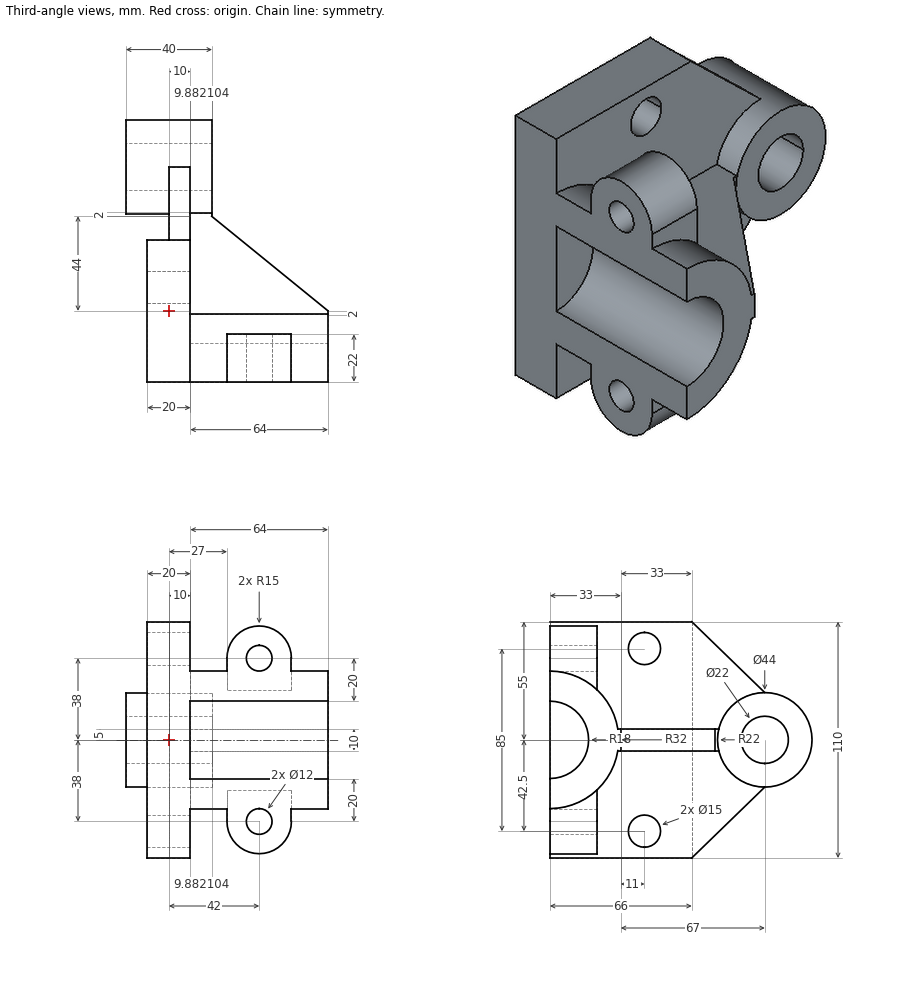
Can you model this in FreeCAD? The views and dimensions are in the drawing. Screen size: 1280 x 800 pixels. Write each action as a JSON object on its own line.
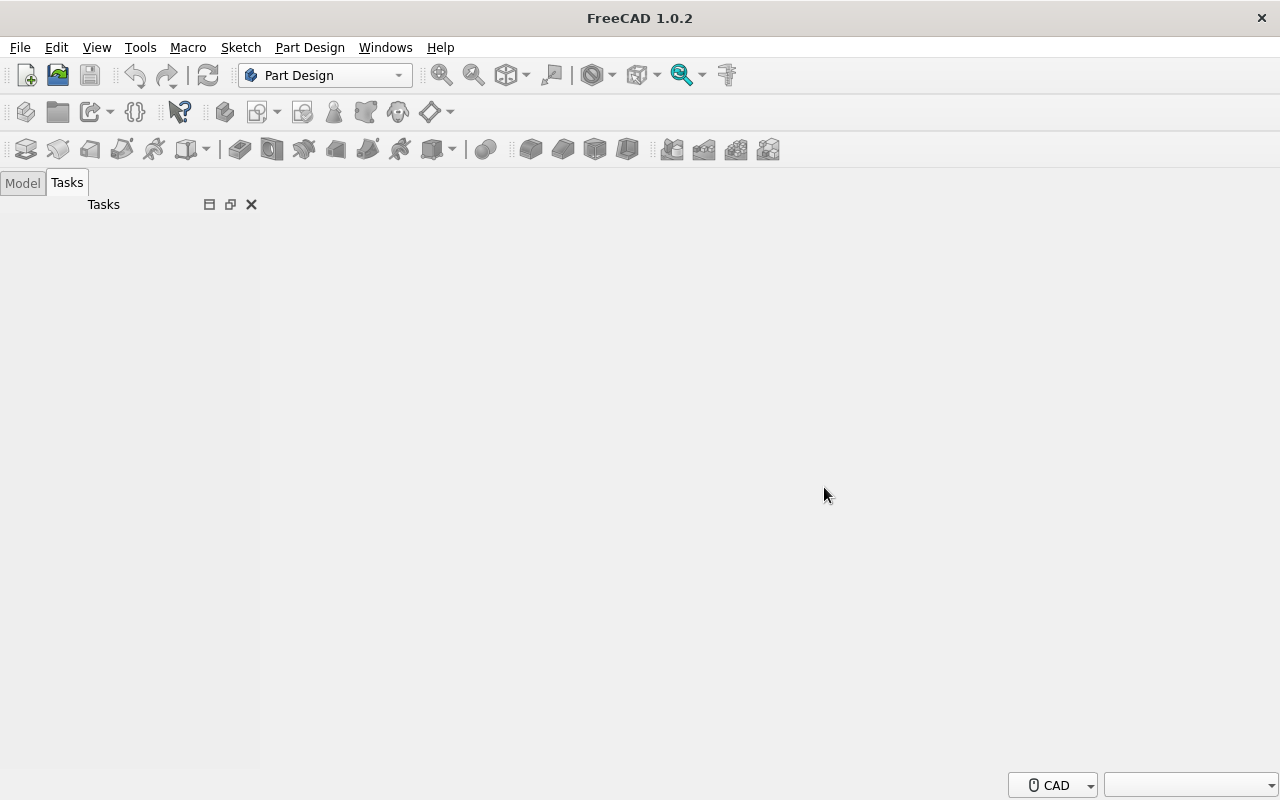
{"action": "left_click", "coordinate": [26, 76]}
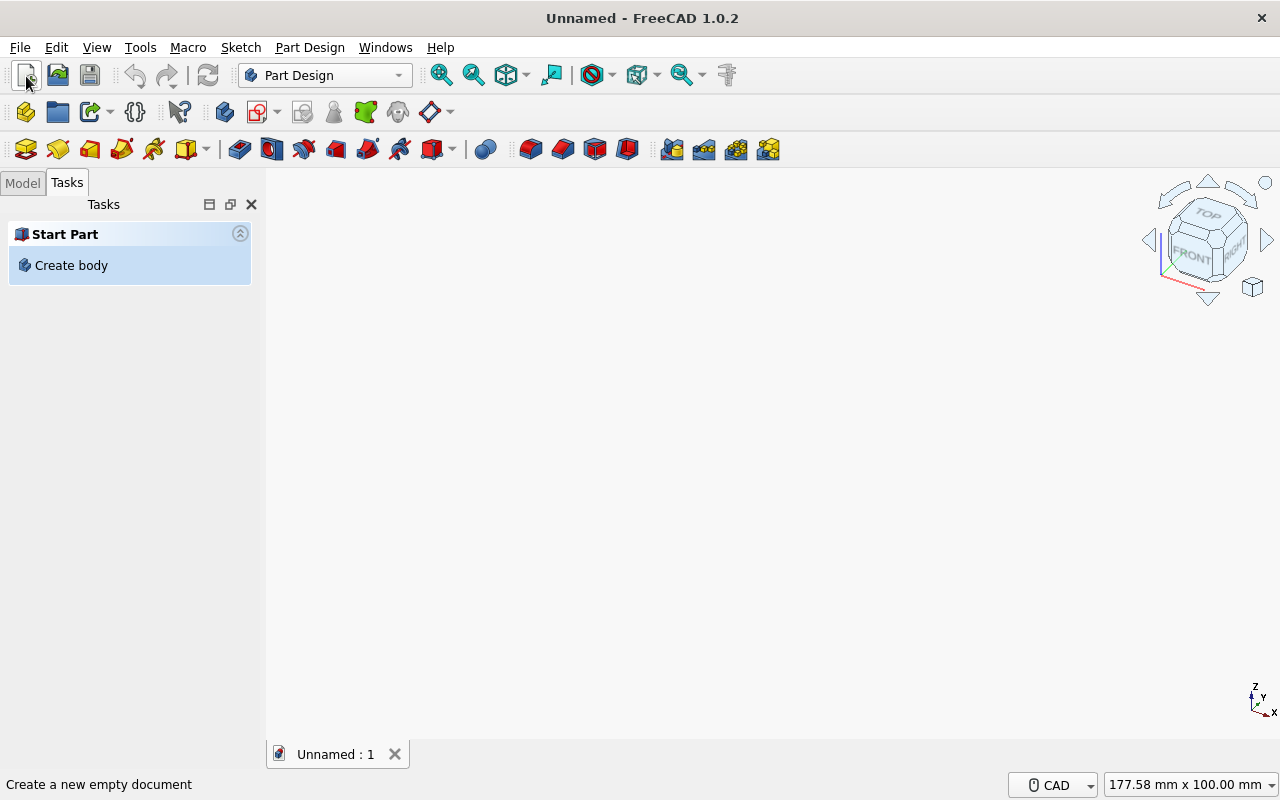
{"action": "left_click", "coordinate": [258, 112]}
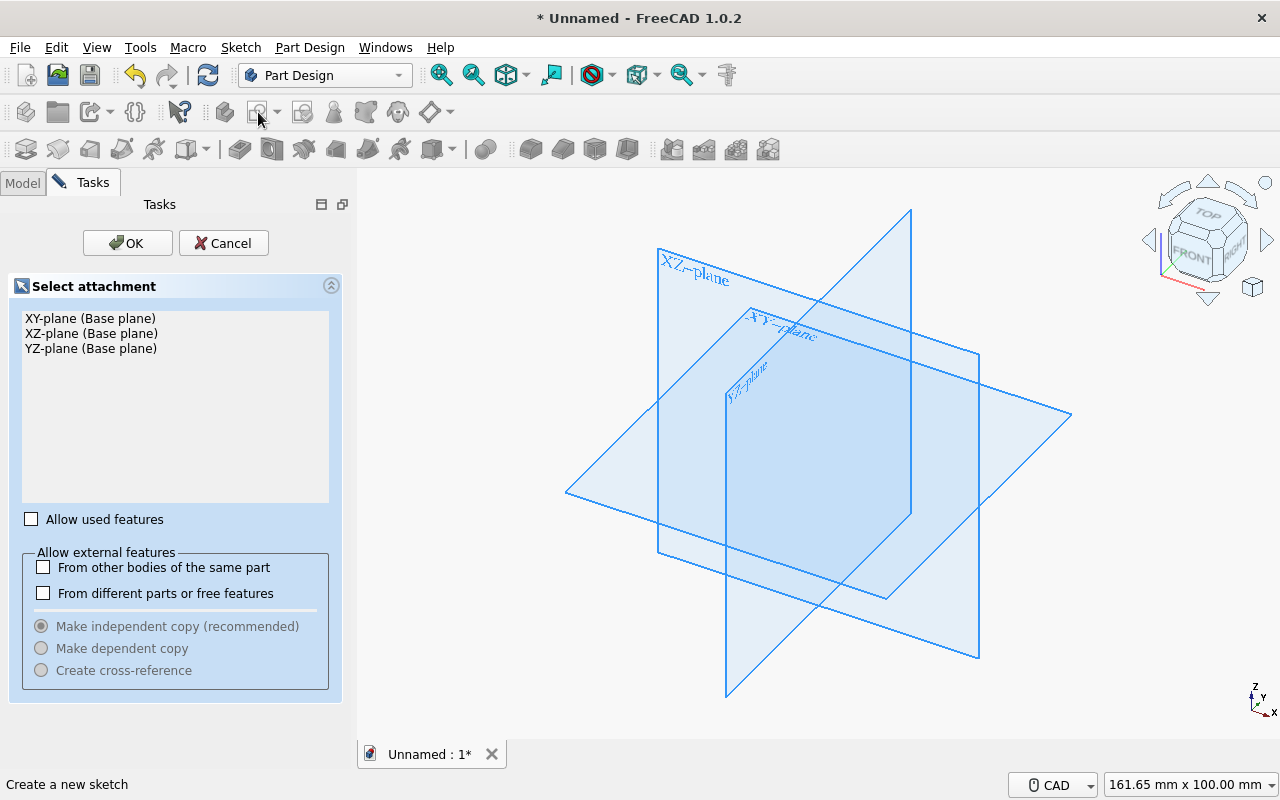
{"action": "left_click", "coordinate": [82, 348]}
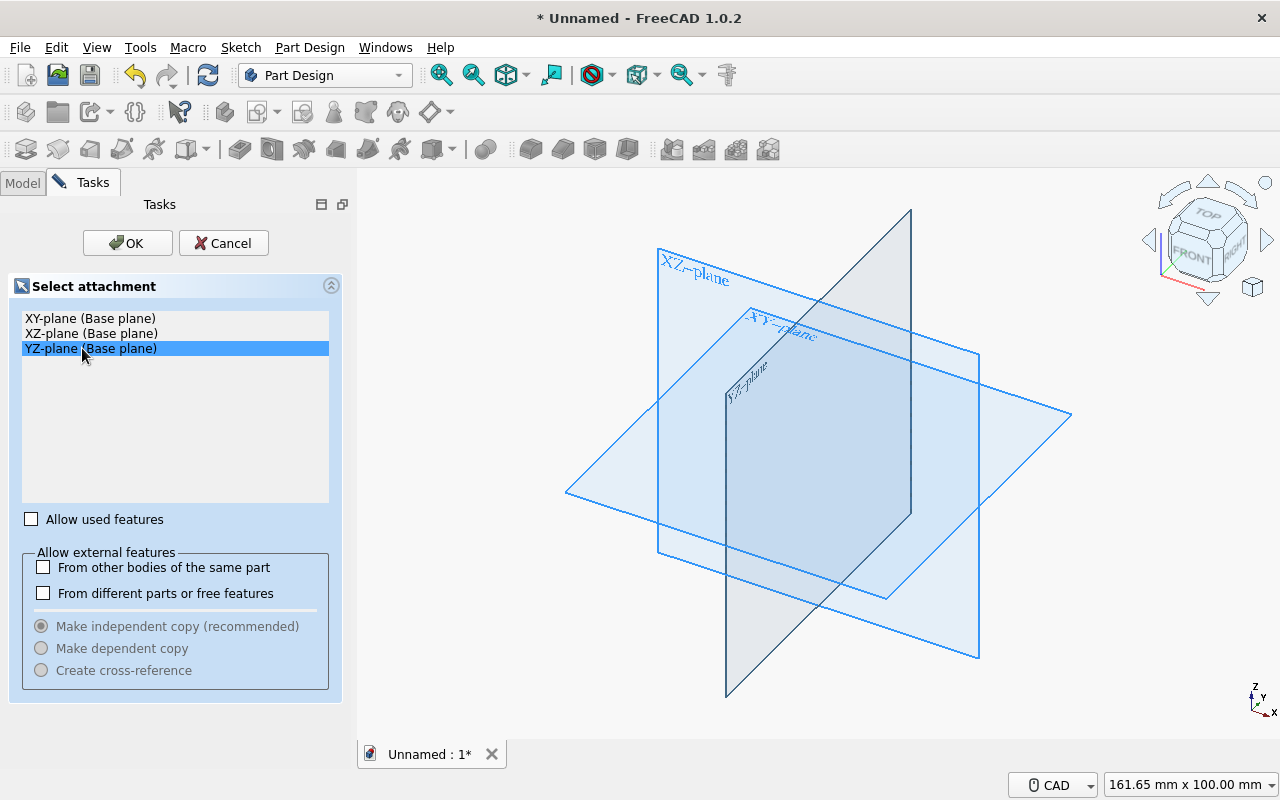
{"action": "left_click", "coordinate": [128, 243]}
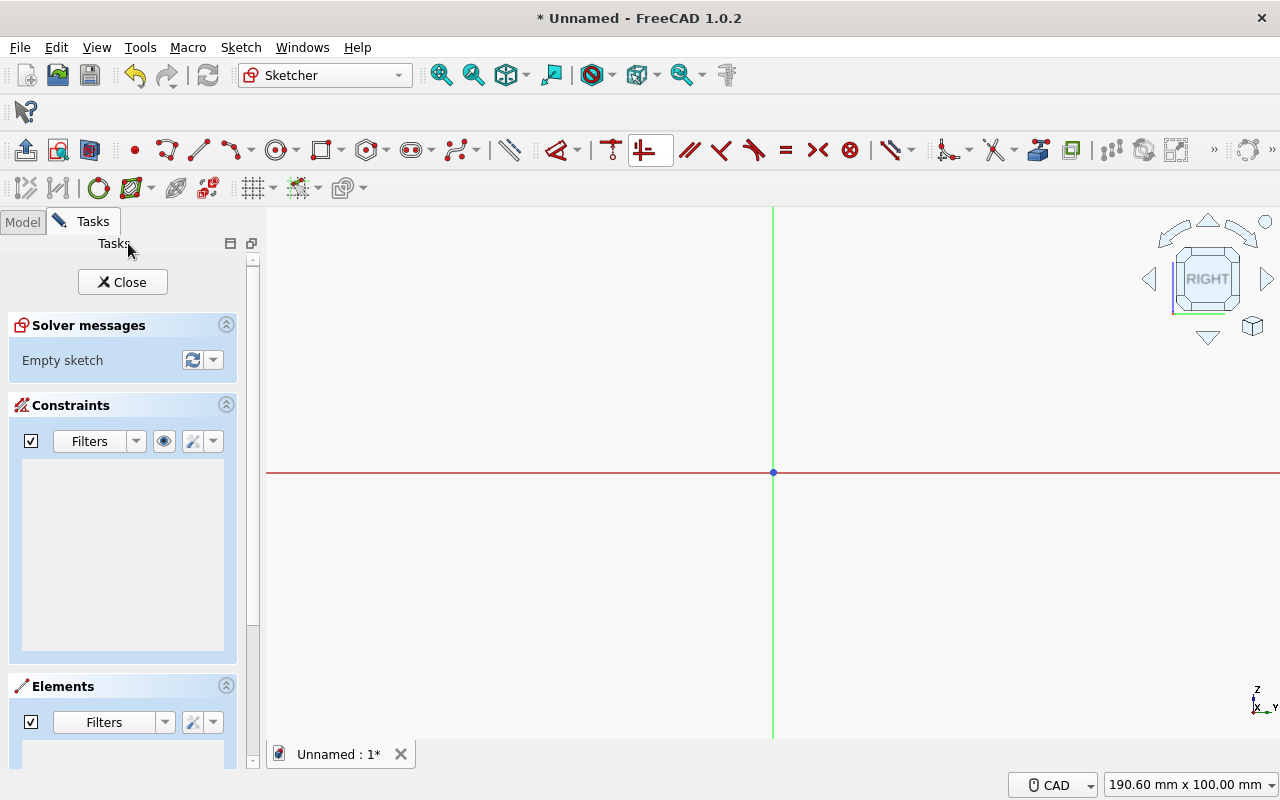
{"action": "scroll", "coordinate": [621, 473], "scroll_direction": "down", "scroll_amount": 3}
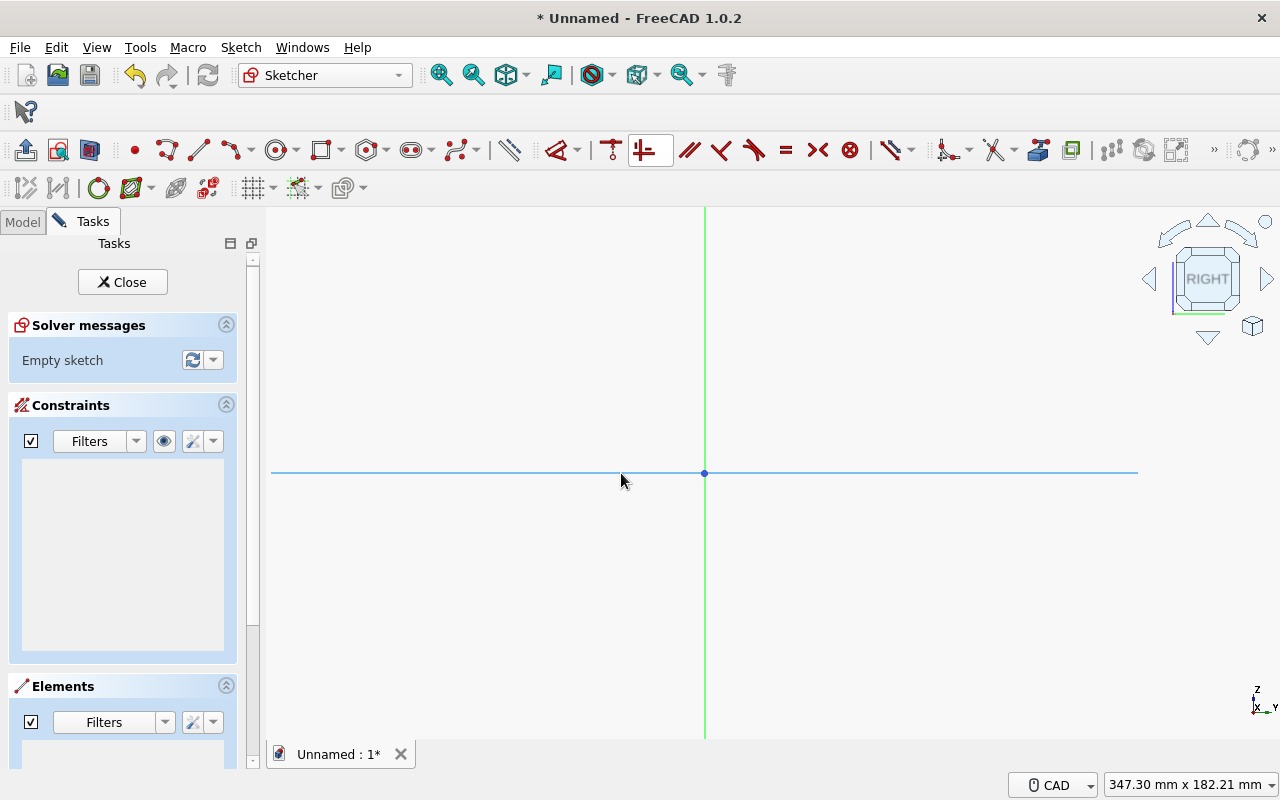
{"action": "key", "text": "g v"}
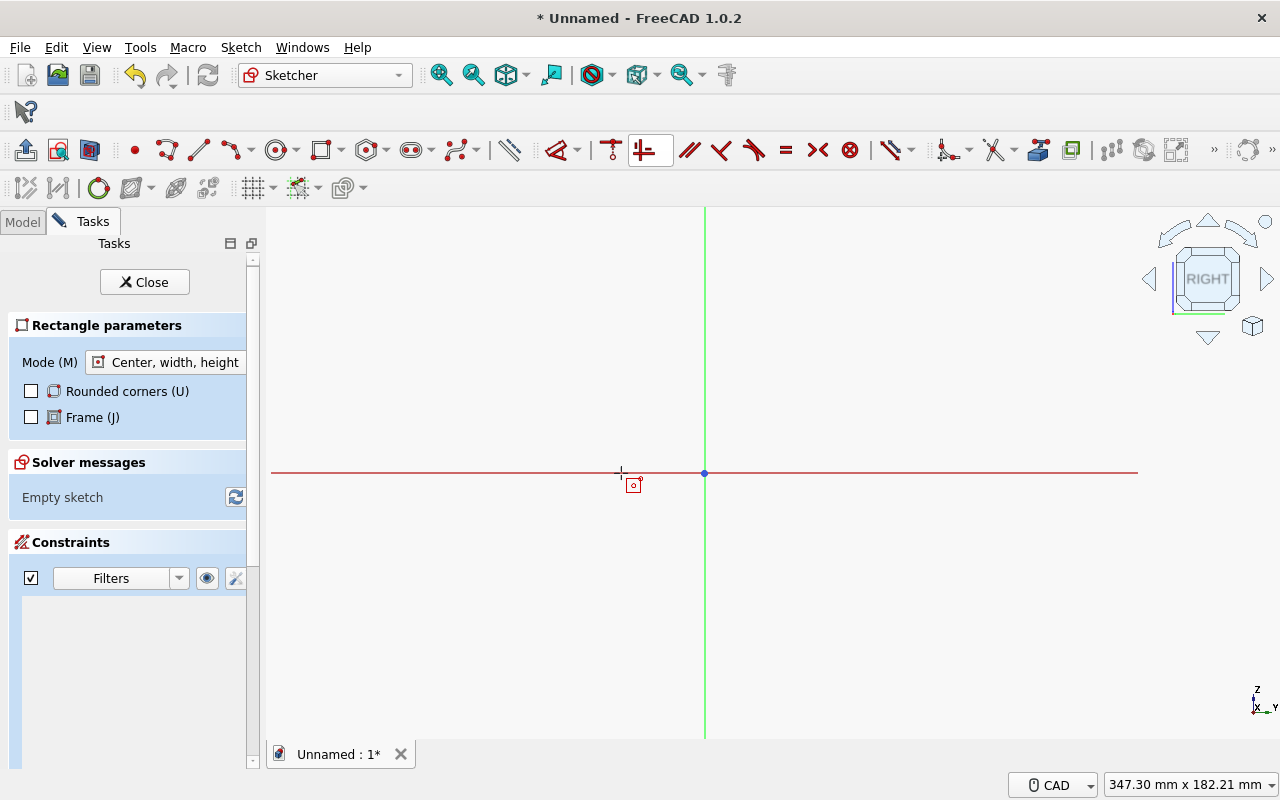
{"action": "left_click", "coordinate": [705, 473]}
{"action": "left_click", "coordinate": [801, 313]}
{"action": "key", "text": "Escape"}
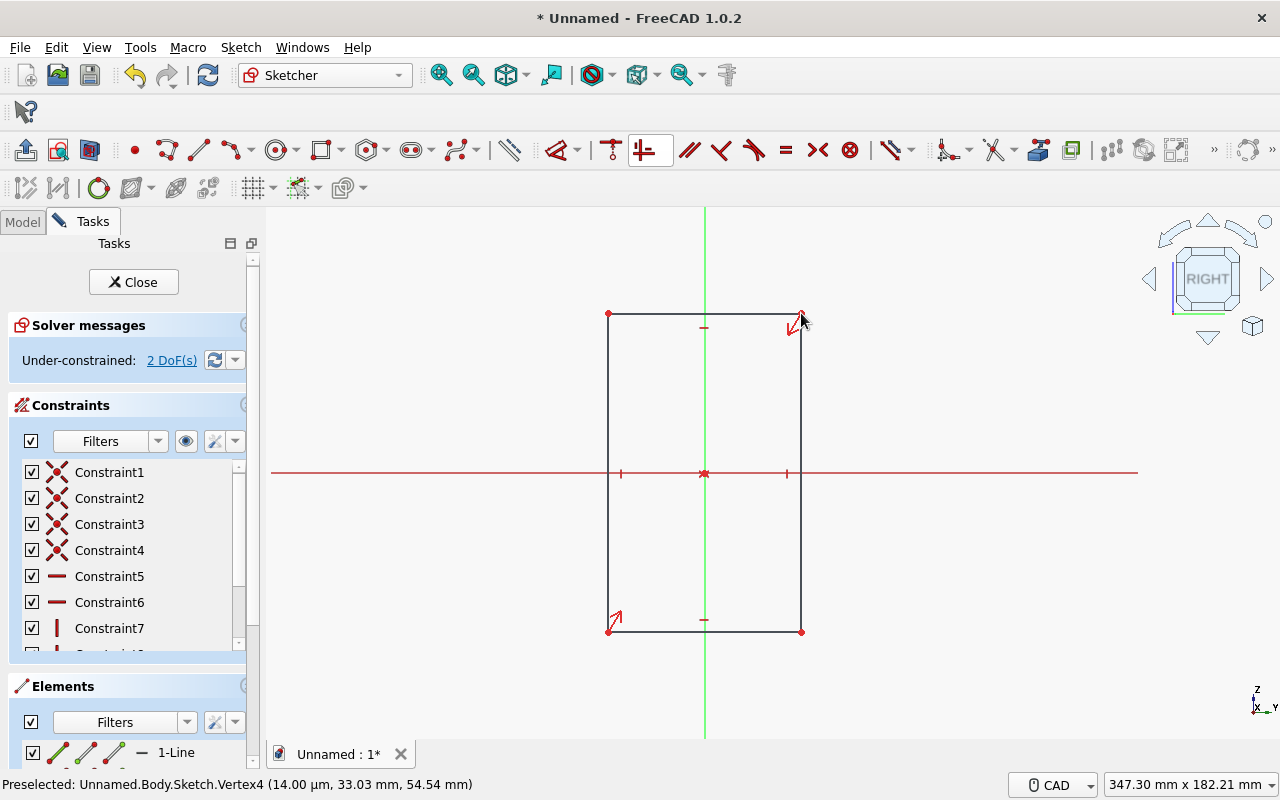
{"action": "left_click", "coordinate": [556, 150]}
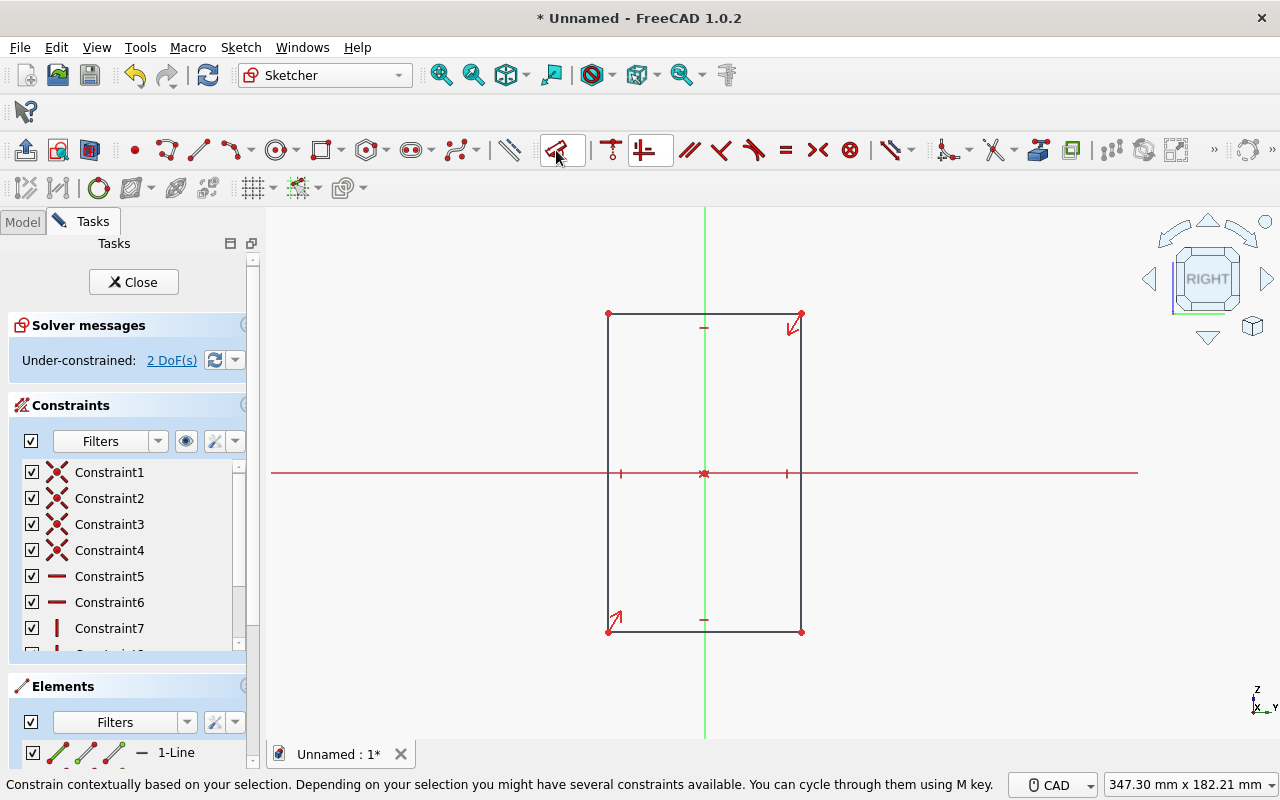
{"action": "left_click", "coordinate": [666, 632]}
{"action": "left_click", "coordinate": [660, 666]}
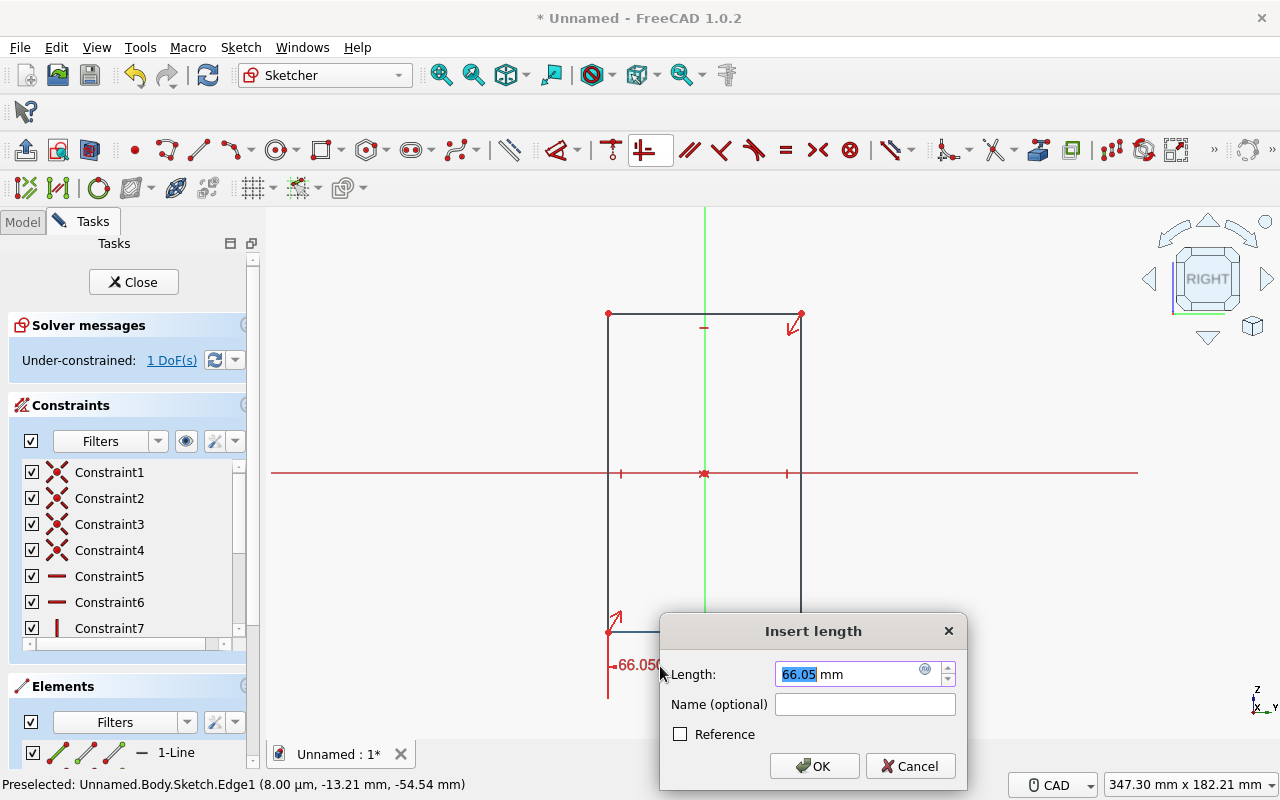
{"action": "type", "text": "66"}
{"action": "key", "text": "Return"}